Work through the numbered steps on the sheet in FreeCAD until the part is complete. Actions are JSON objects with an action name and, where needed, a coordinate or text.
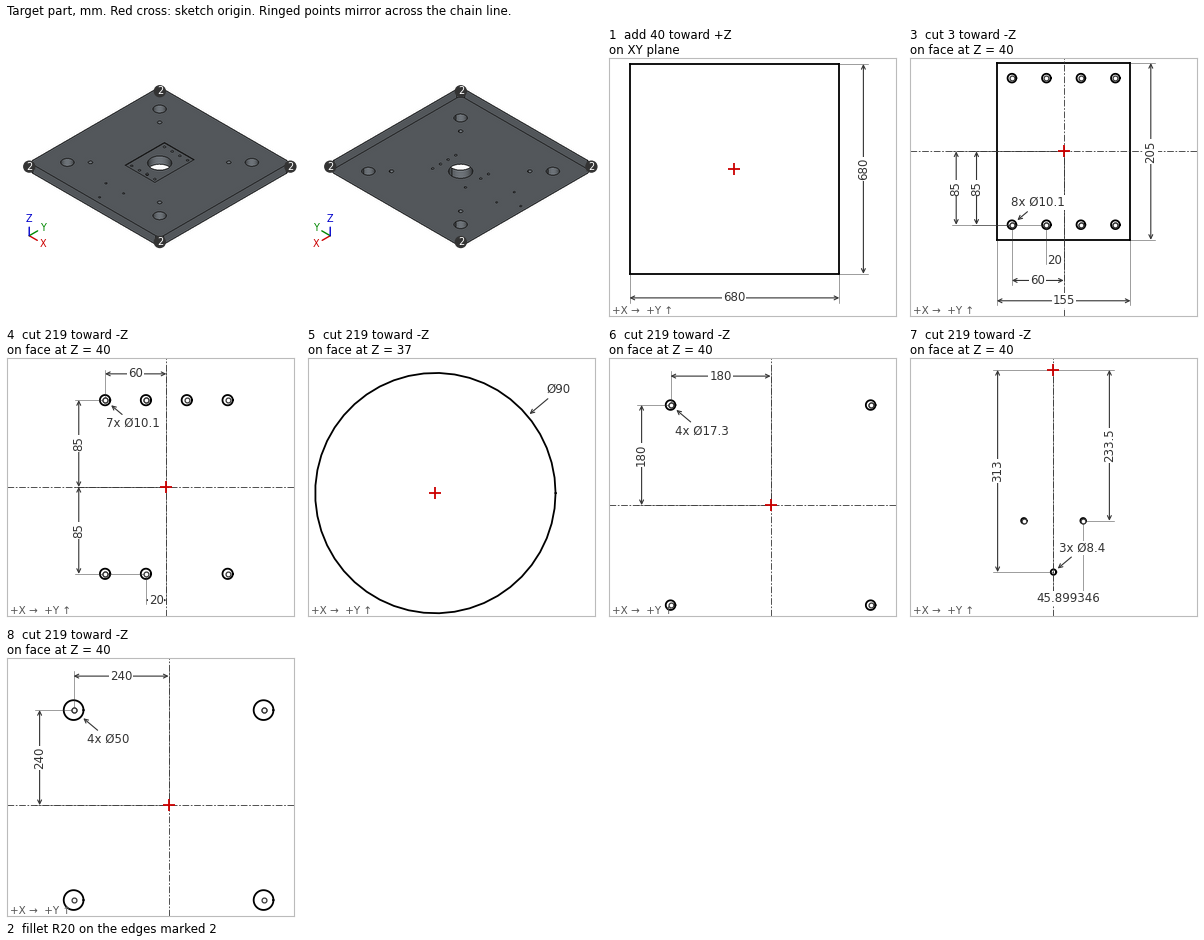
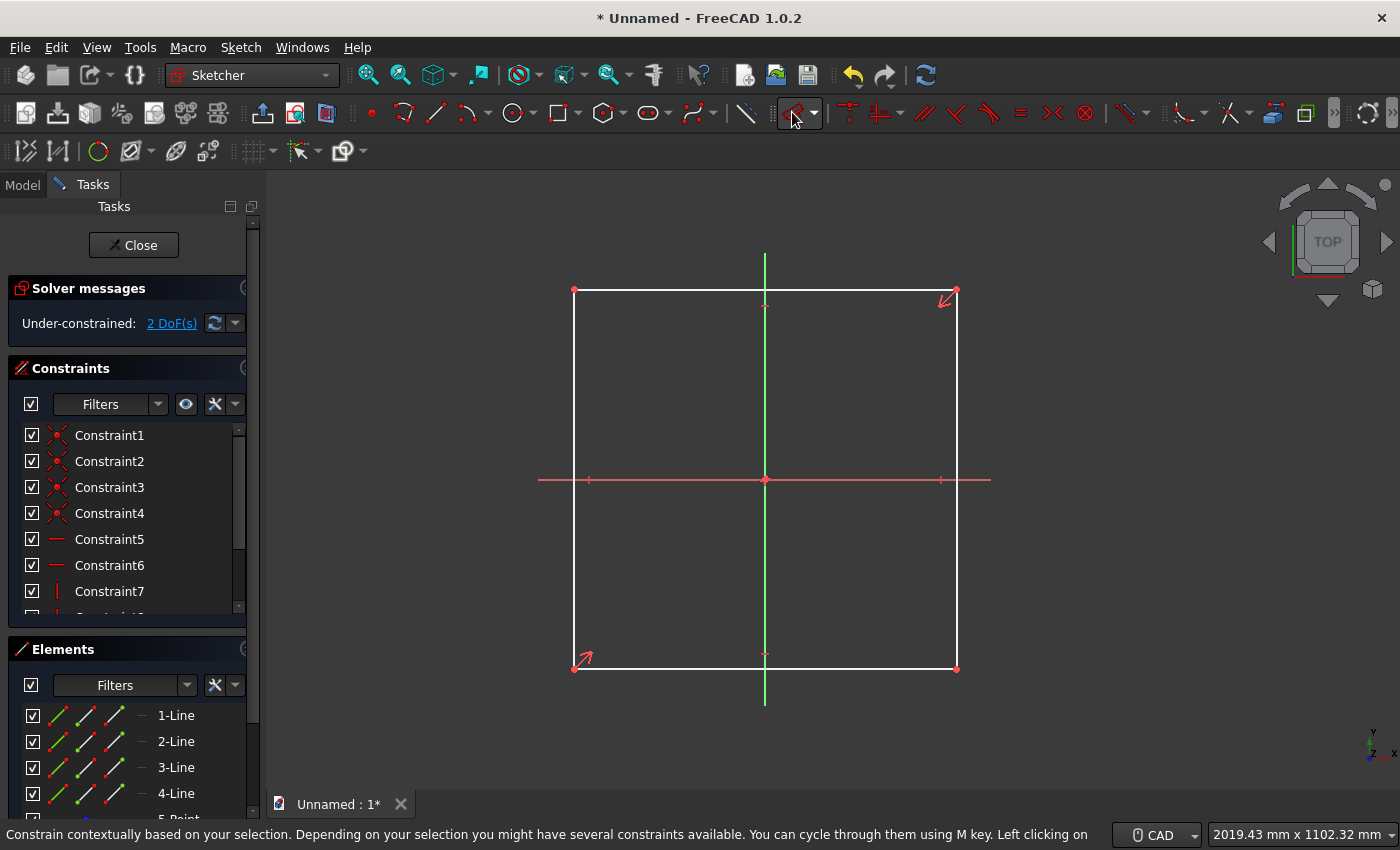
{"action": "left_click", "coordinate": [689, 669]}
{"action": "left_click", "coordinate": [677, 703]}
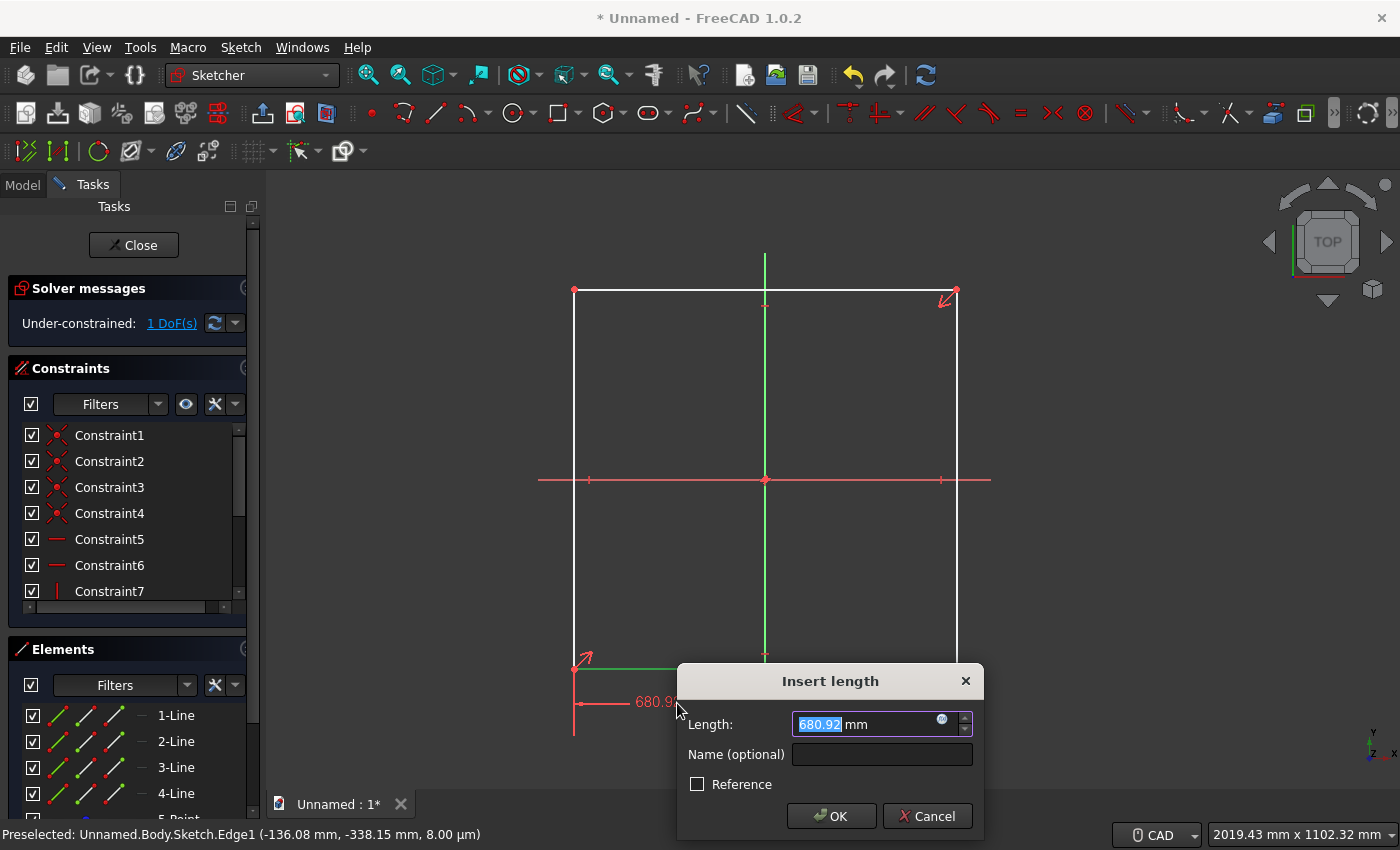
{"action": "type", "text": "680"}
{"action": "key", "text": "Return"}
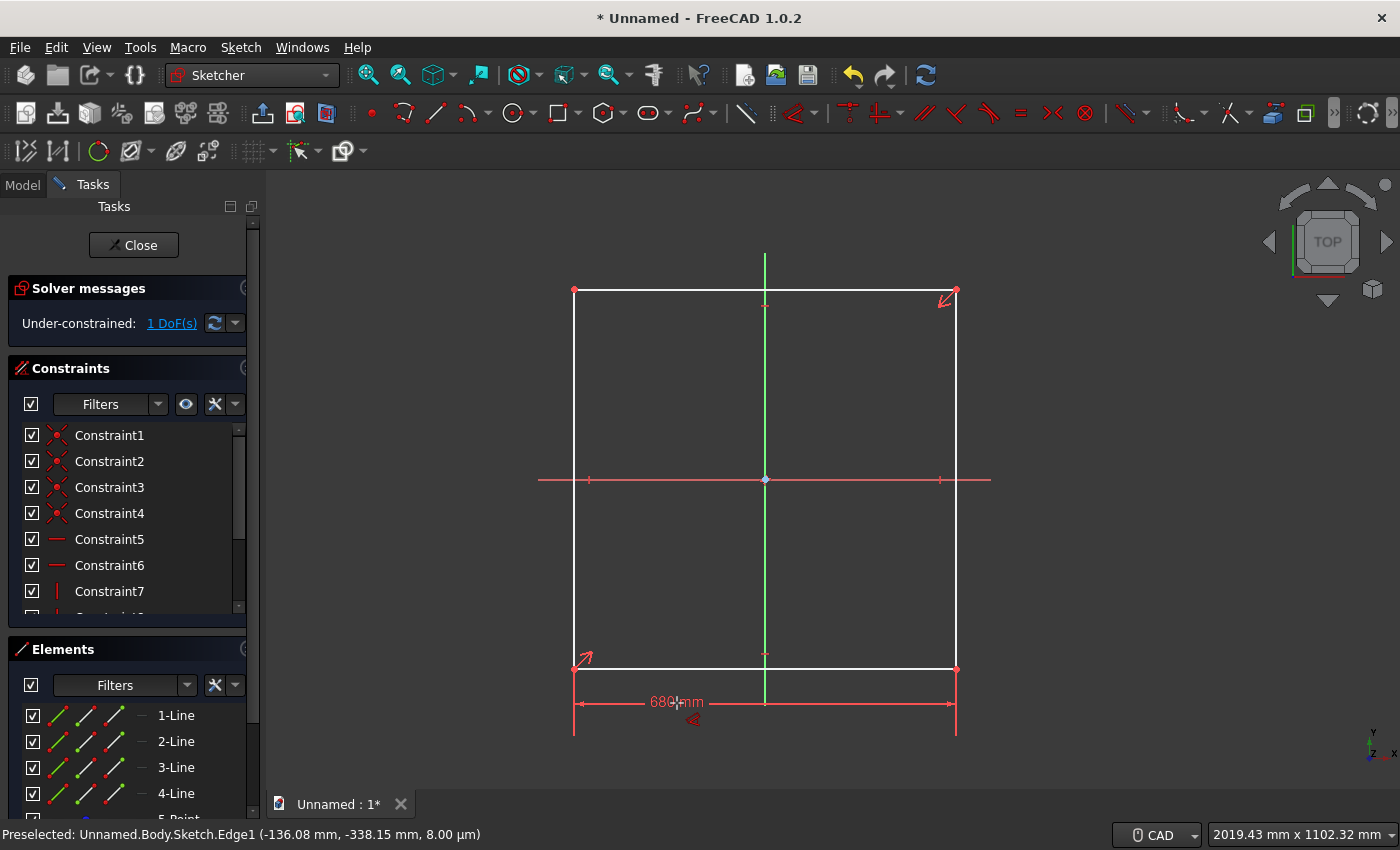
{"action": "left_click", "coordinate": [956, 555]}
{"action": "left_click", "coordinate": [990, 392]}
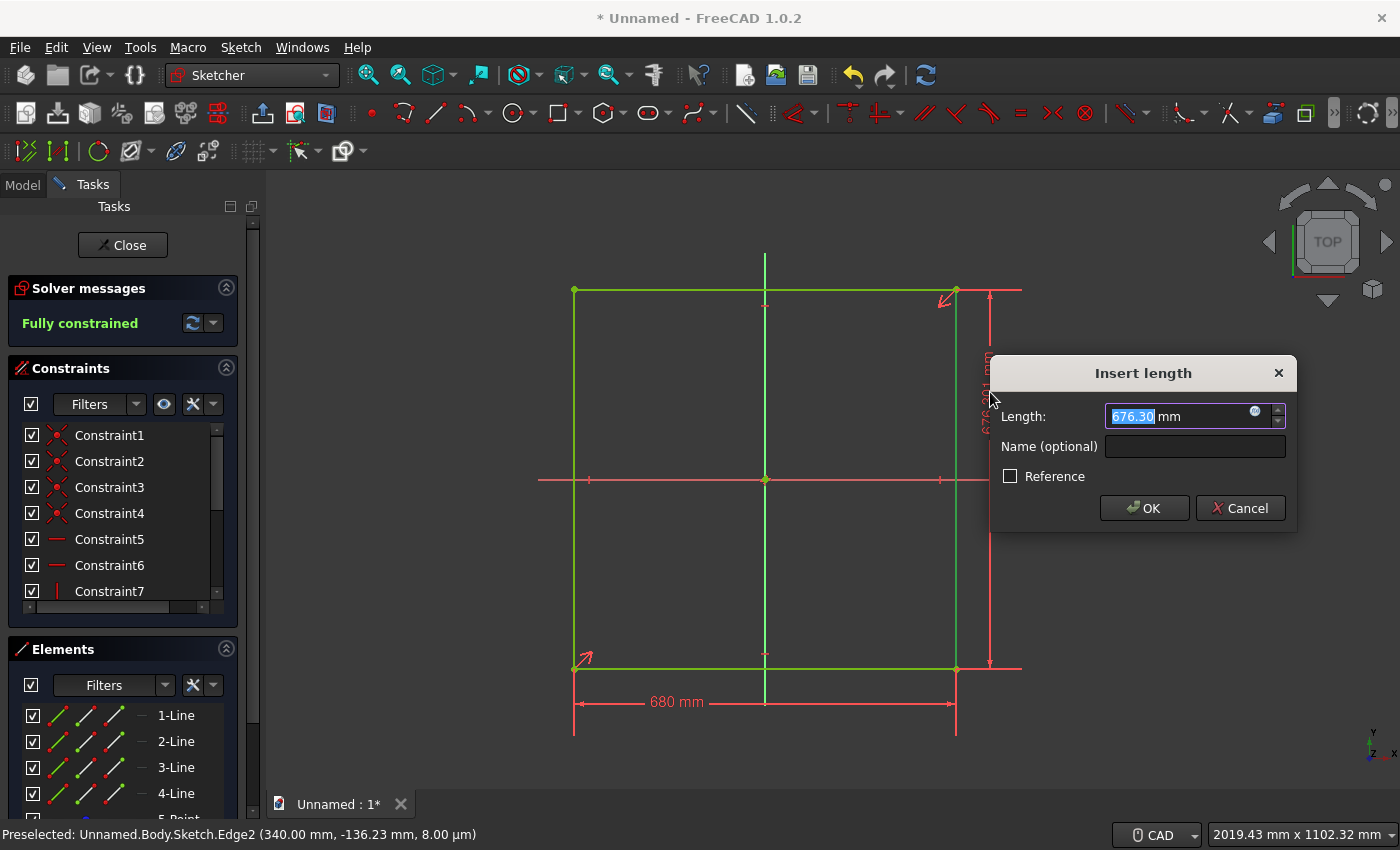
{"action": "type", "text": "680"}
{"action": "key", "text": "Return"}
{"action": "key", "text": "Escape"}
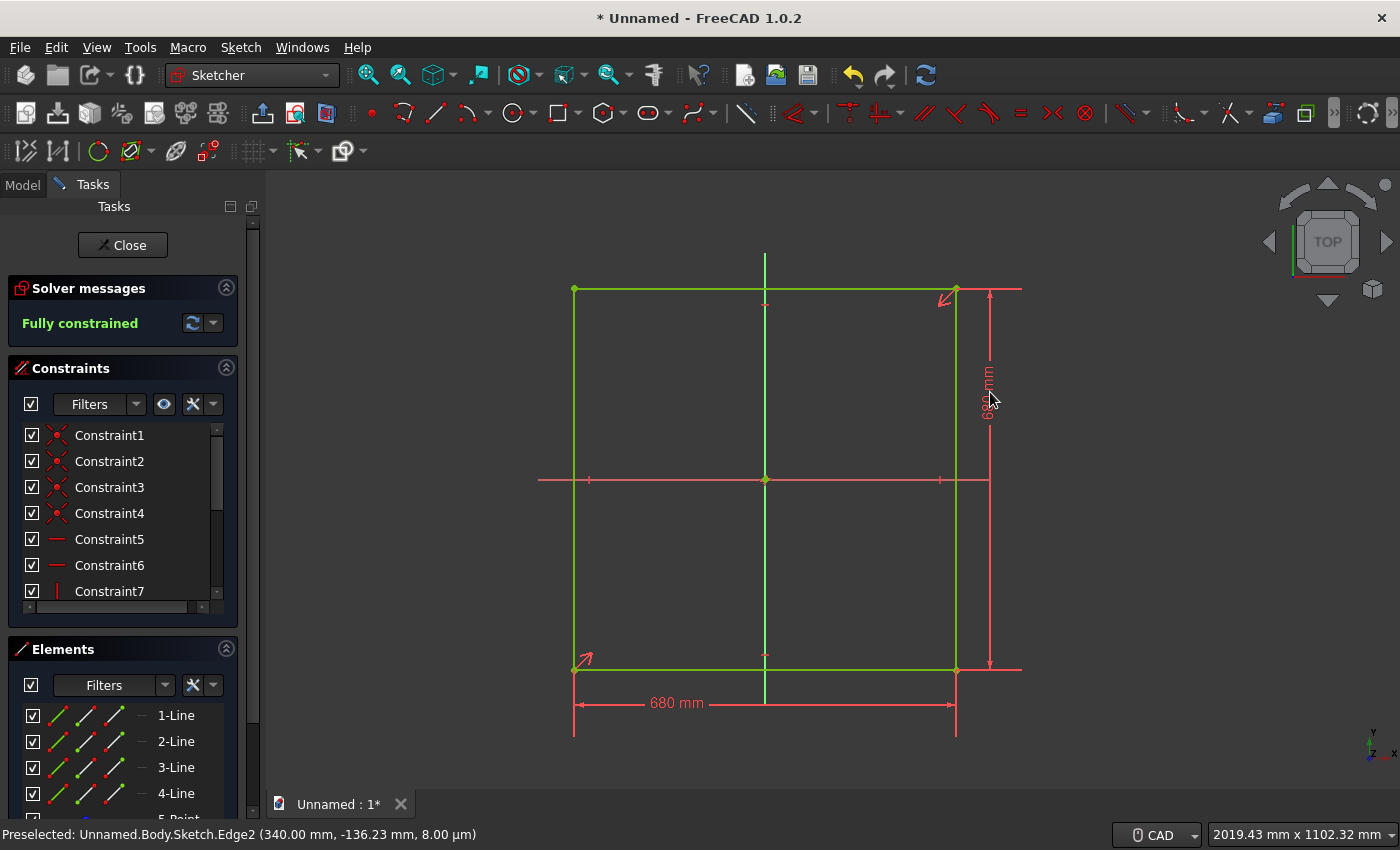
{"action": "left_click", "coordinate": [123, 245]}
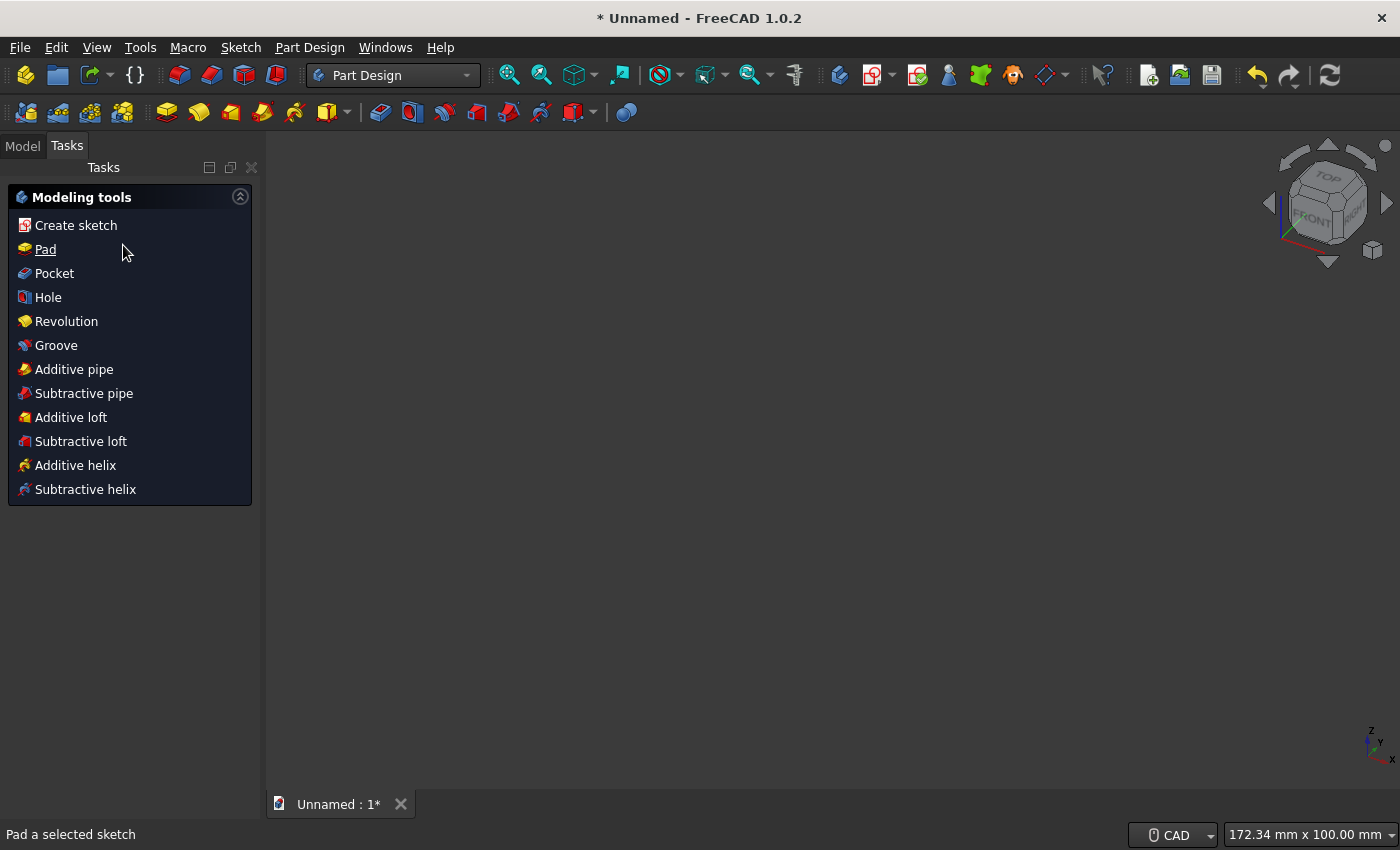
{"action": "left_click", "coordinate": [168, 112]}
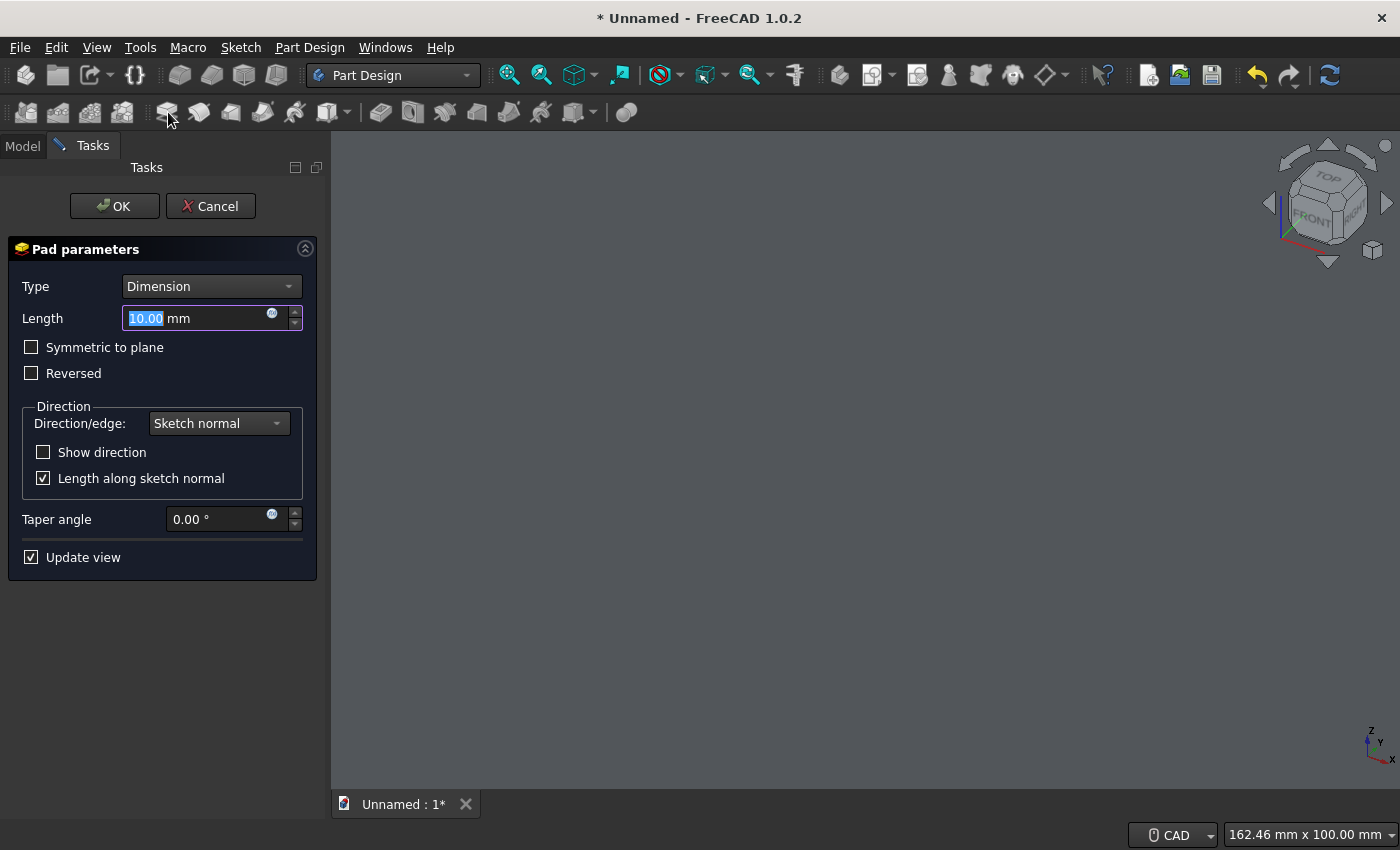
{"action": "type", "text": "40"}
{"action": "key", "text": "Tab"}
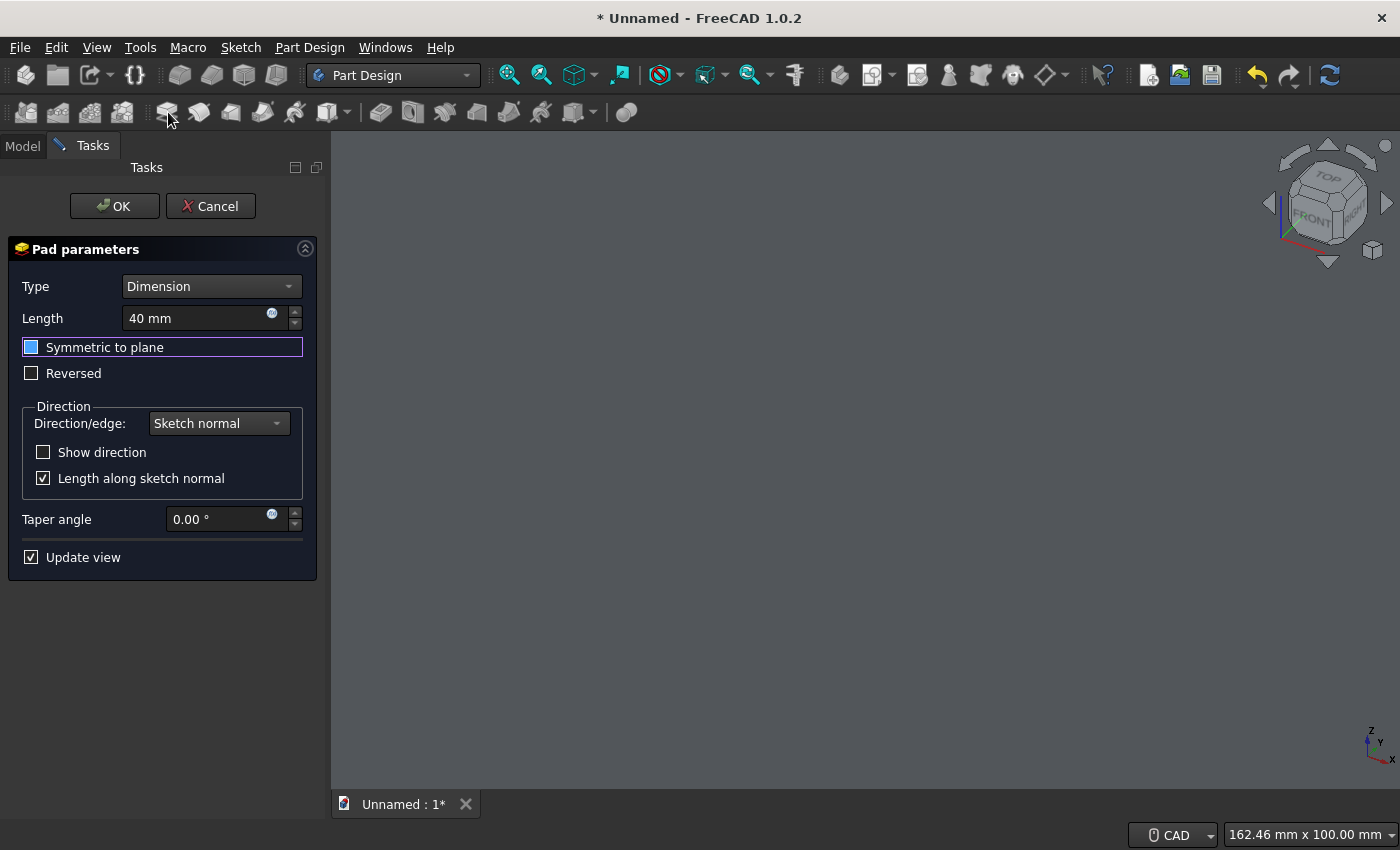
{"action": "left_click", "coordinate": [115, 206]}